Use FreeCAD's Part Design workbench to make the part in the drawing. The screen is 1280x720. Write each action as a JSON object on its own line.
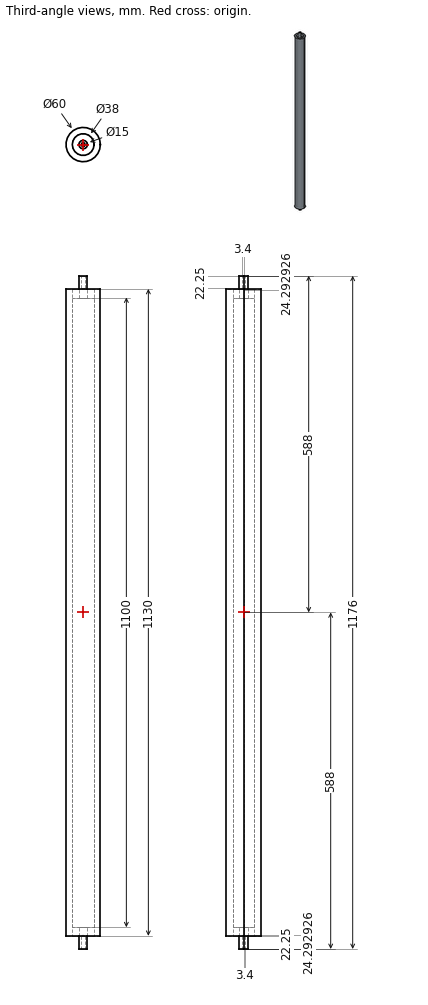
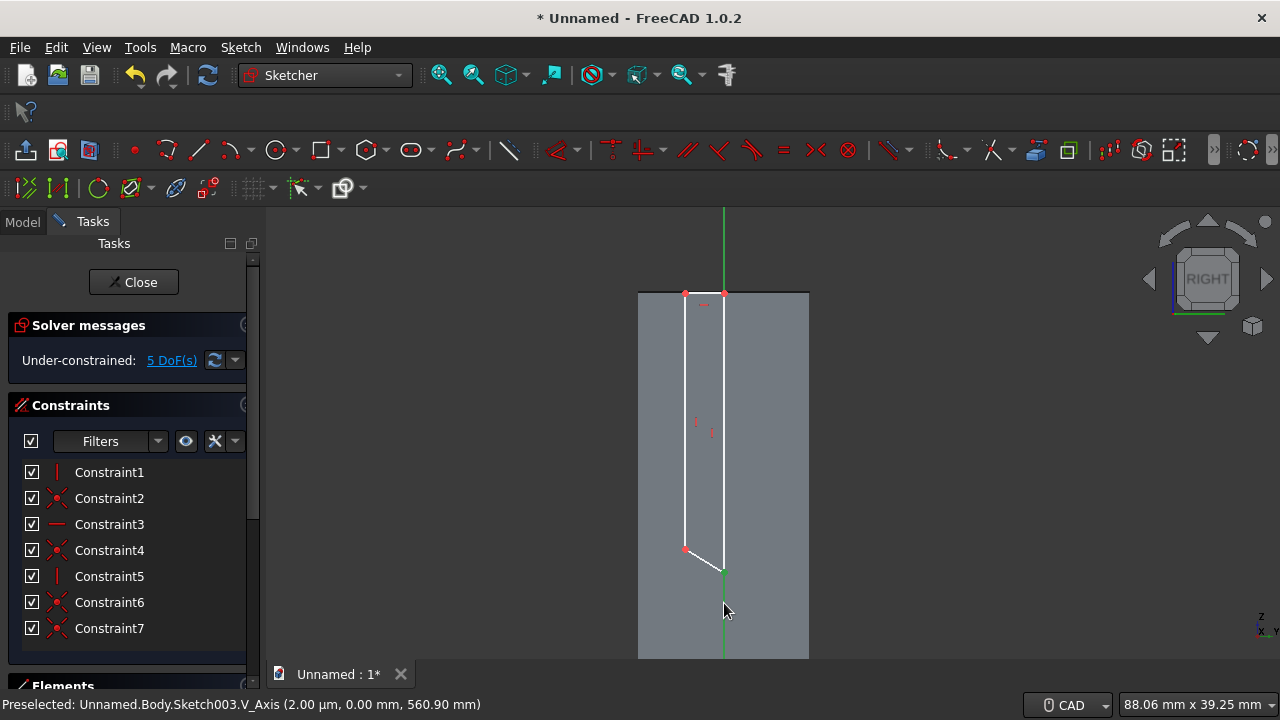
{"action": "left_click", "coordinate": [612, 150]}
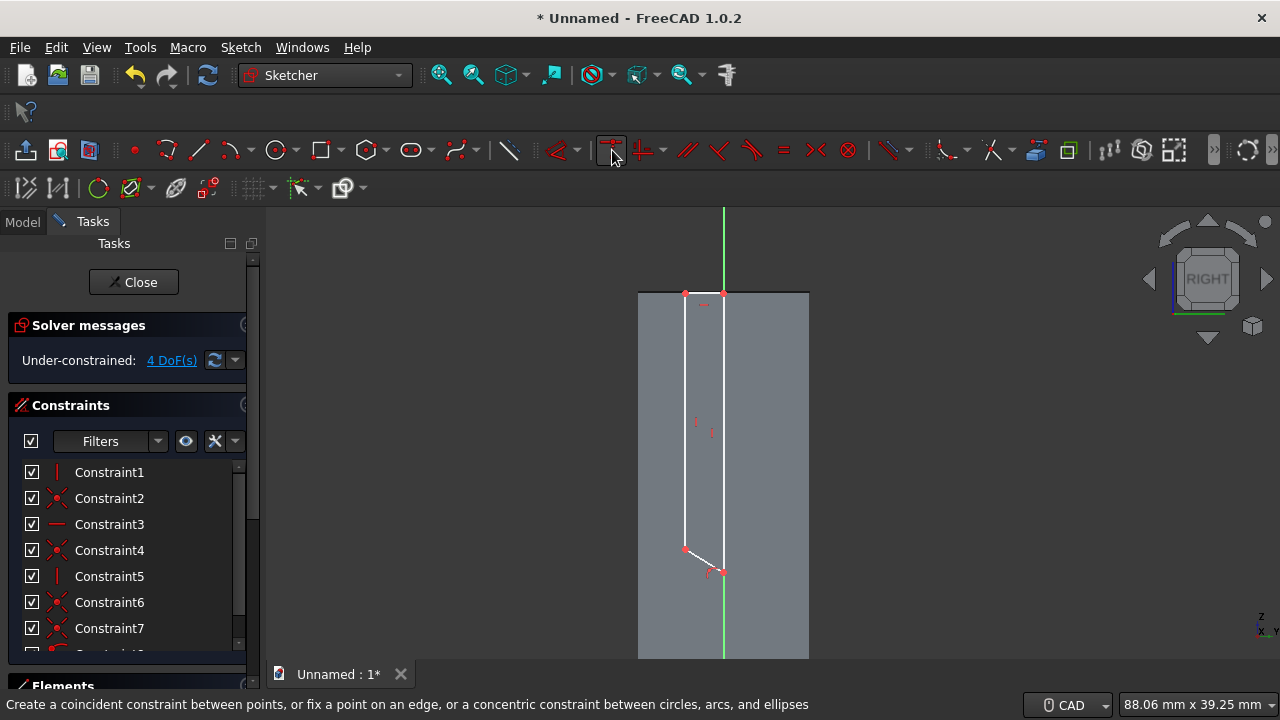
{"action": "key", "text": "d"}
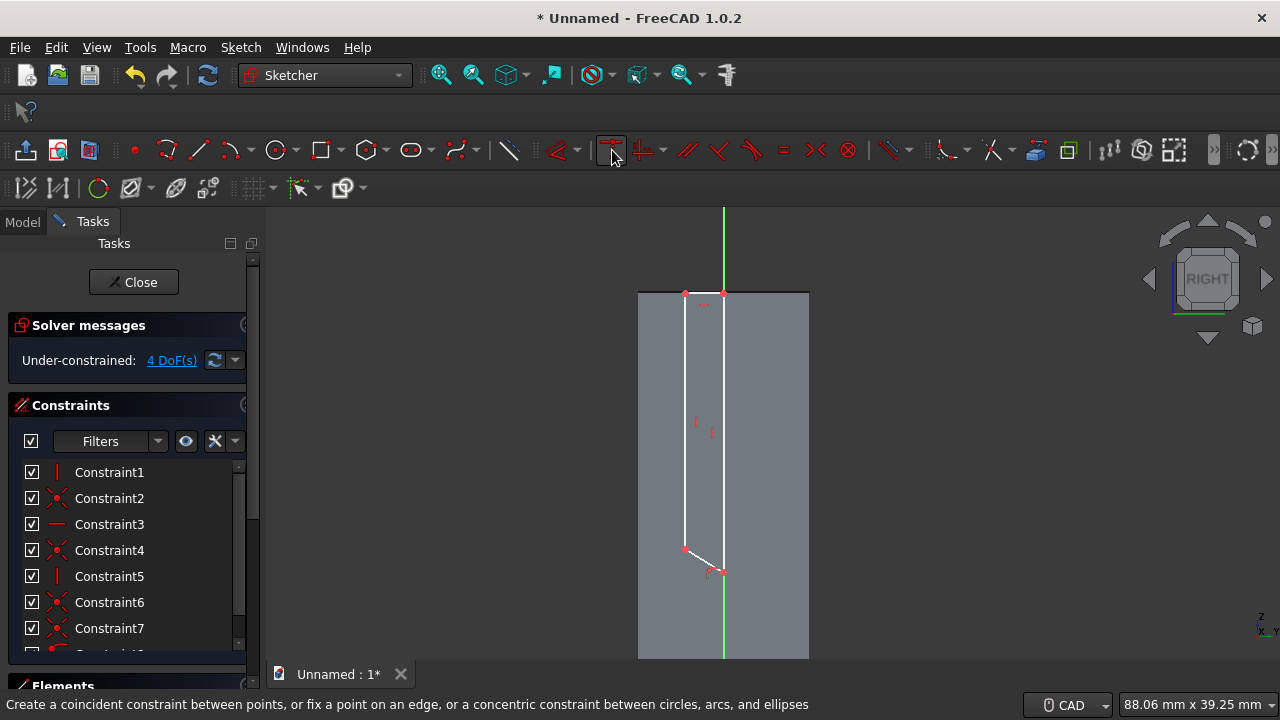
{"action": "left_click", "coordinate": [712, 293]}
{"action": "left_click", "coordinate": [704, 259]}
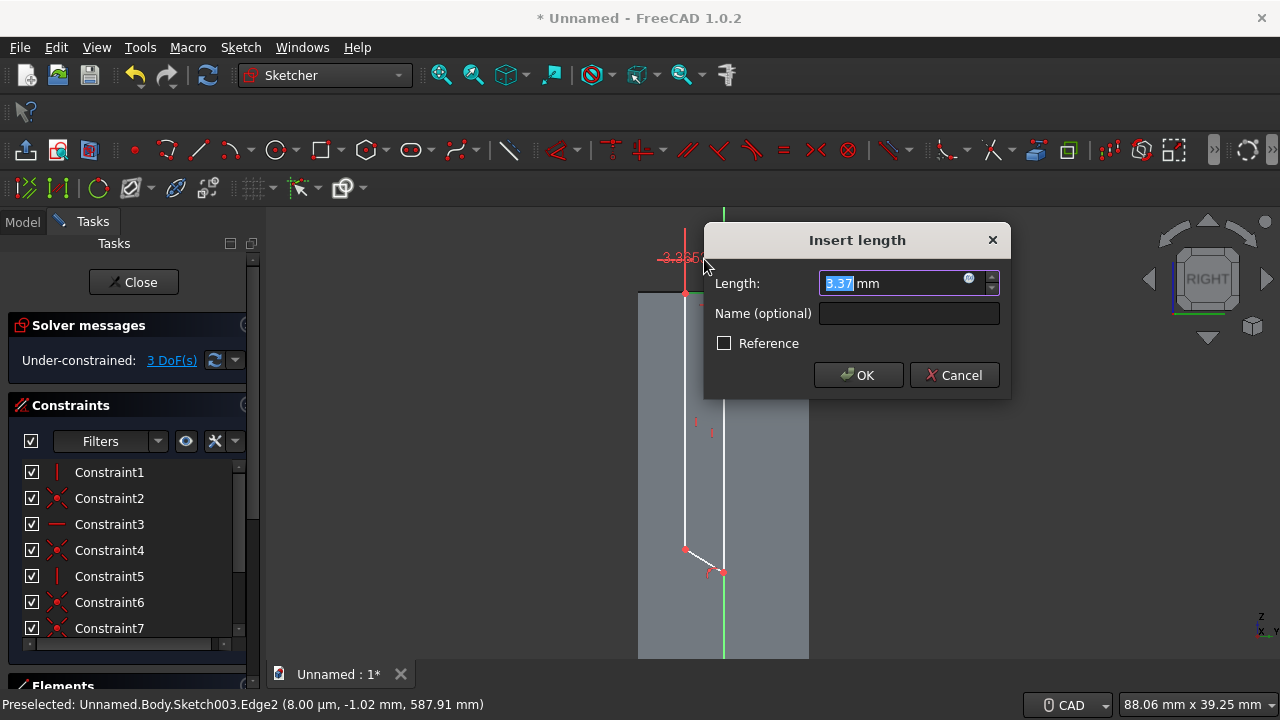
{"action": "type", "text": "3.4"}
{"action": "key", "text": "Return"}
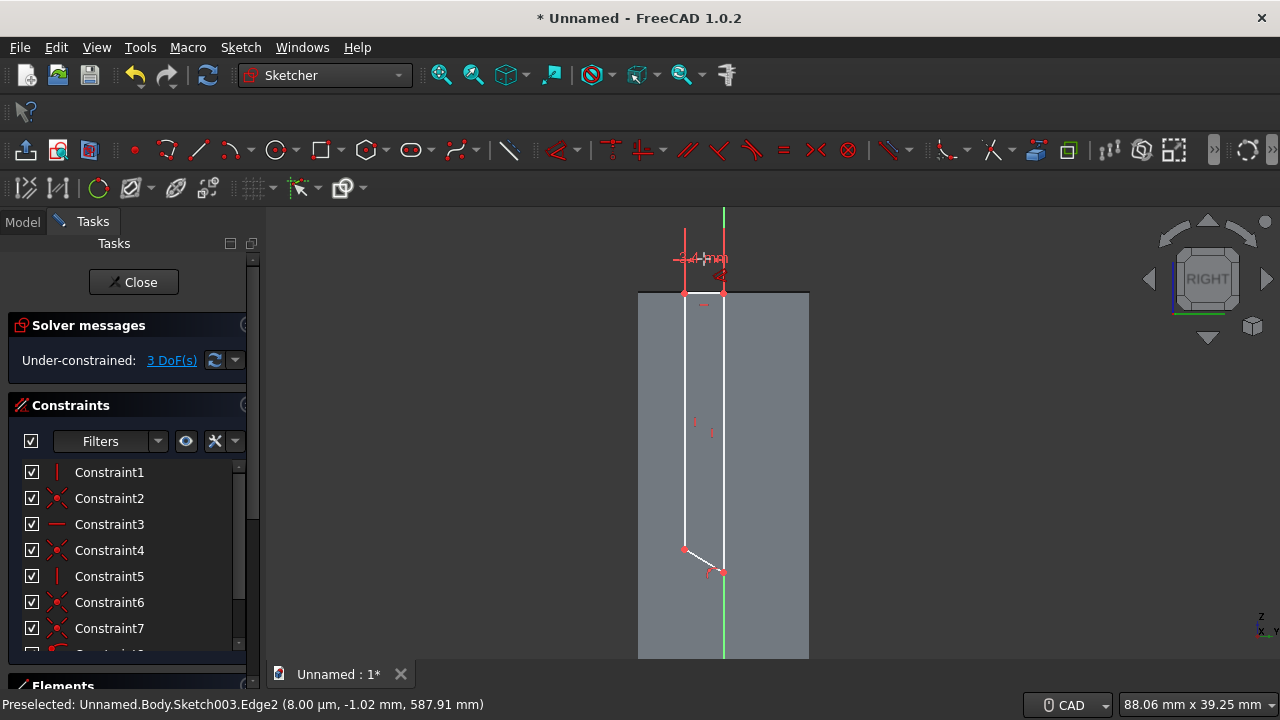
{"action": "left_click", "coordinate": [724, 293]}
{"action": "left_click", "coordinate": [758, 462]}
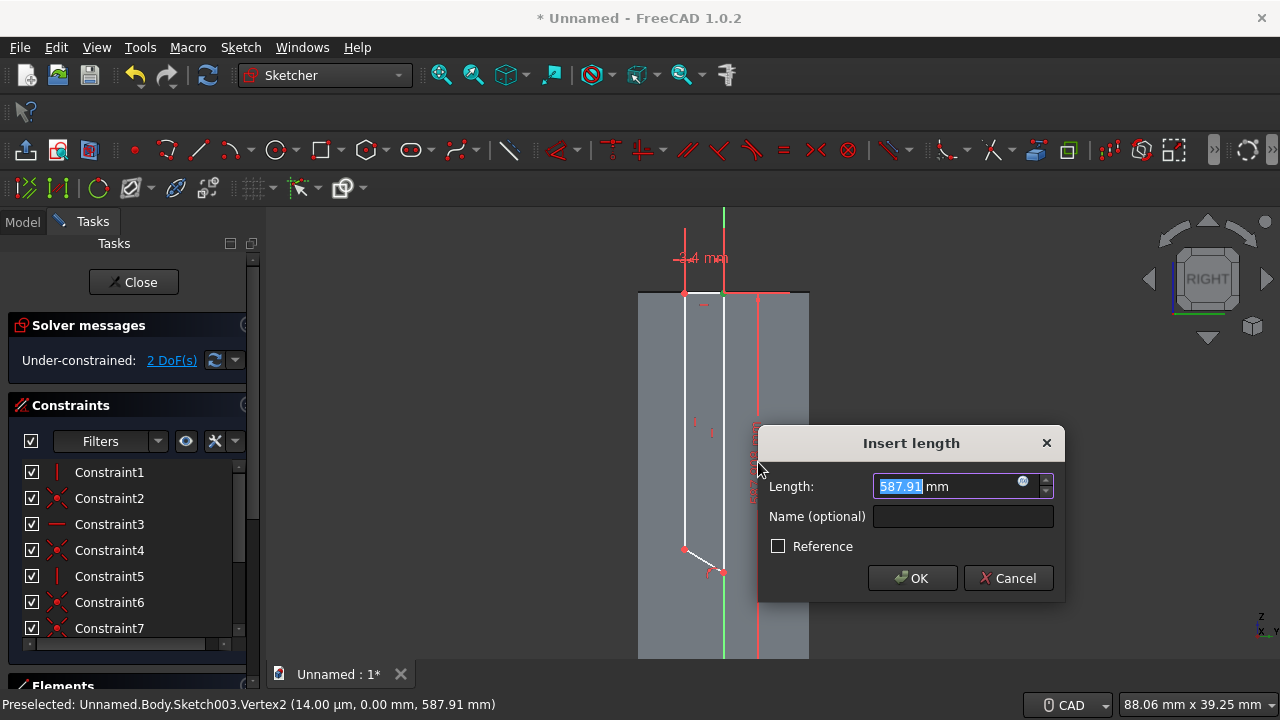
{"action": "type", "text": "588"}
{"action": "key", "text": "Return"}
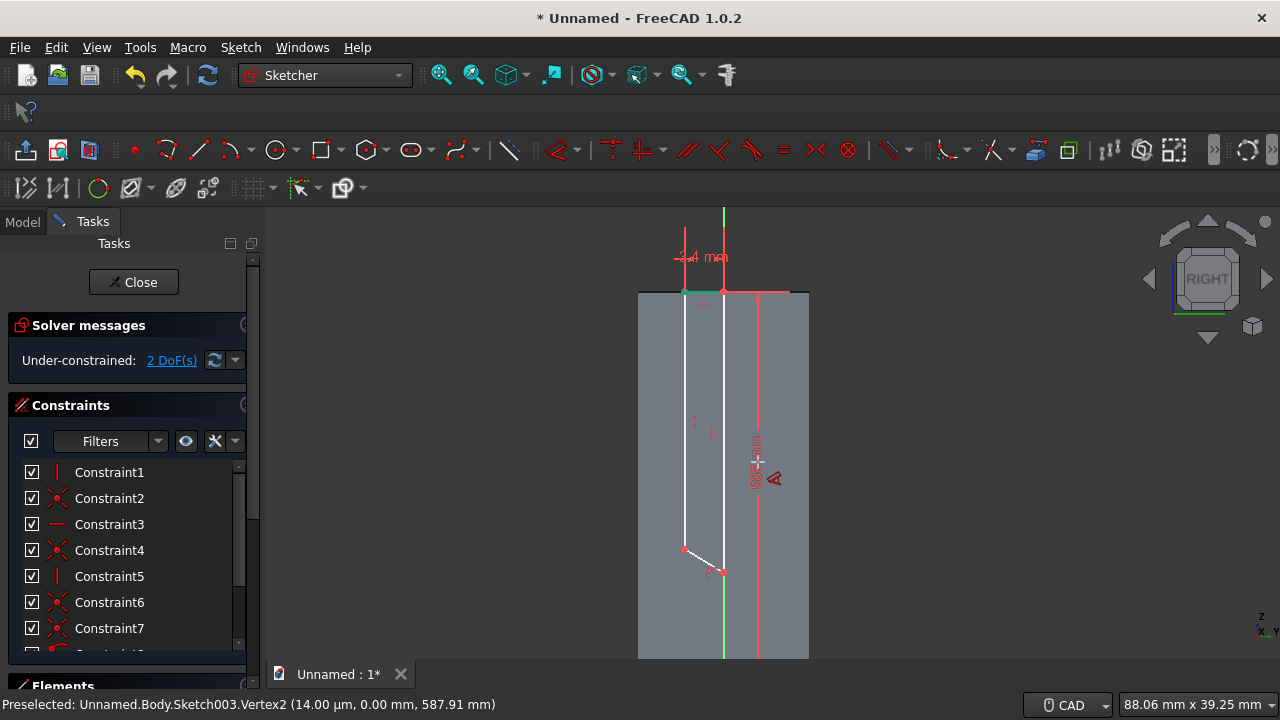
{"action": "left_click", "coordinate": [685, 369]}
{"action": "left_click", "coordinate": [651, 420]}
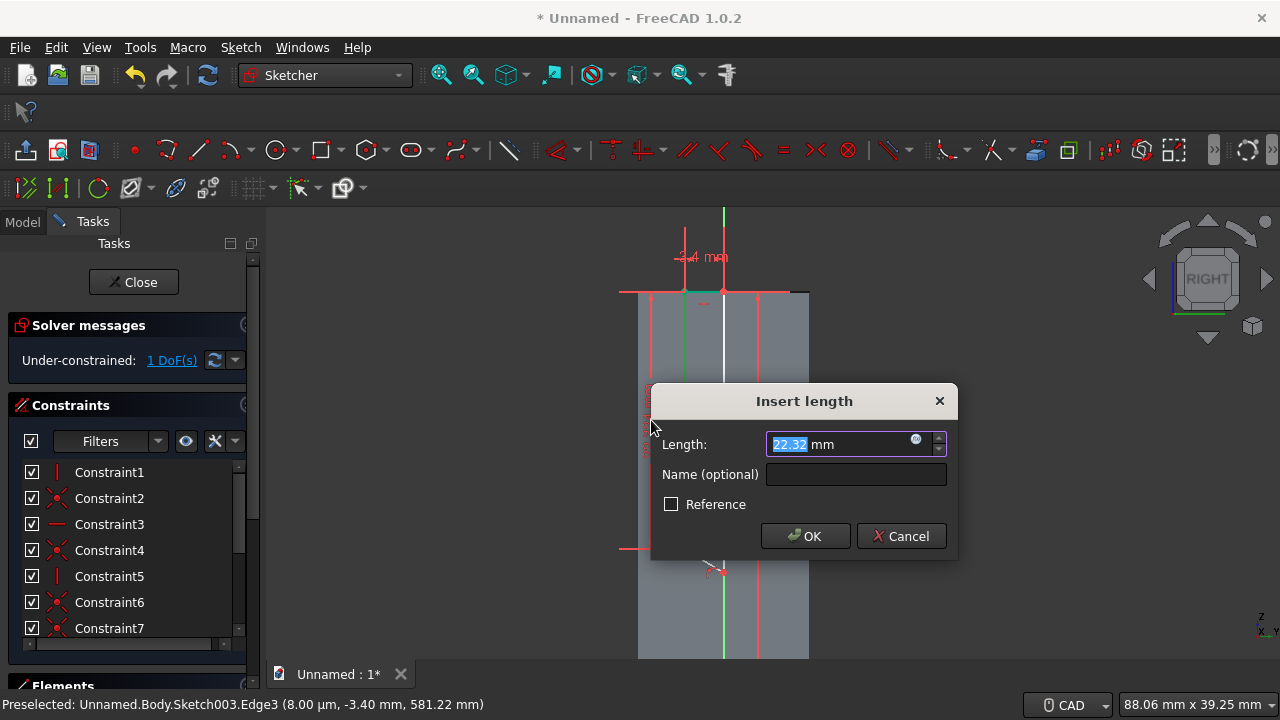
{"action": "type", "text": "22.25"}
{"action": "key", "text": "Return"}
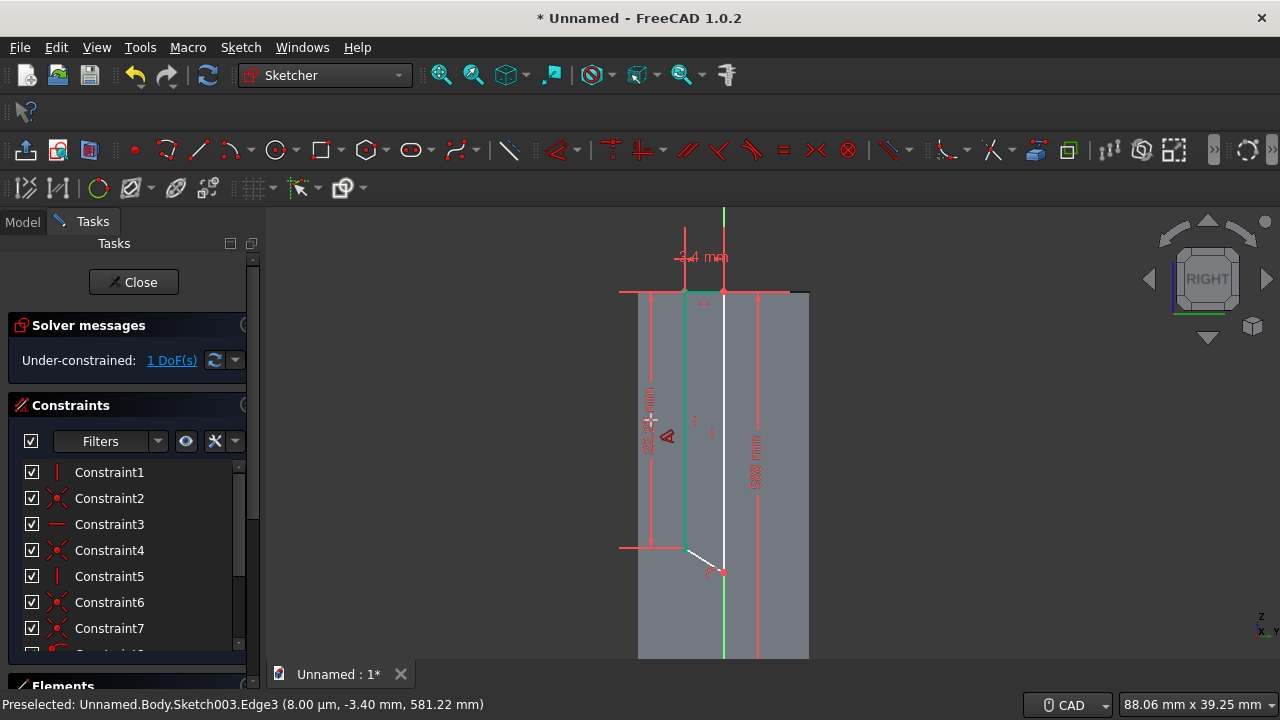
{"action": "left_click", "coordinate": [724, 489]}
{"action": "left_click", "coordinate": [758, 432]}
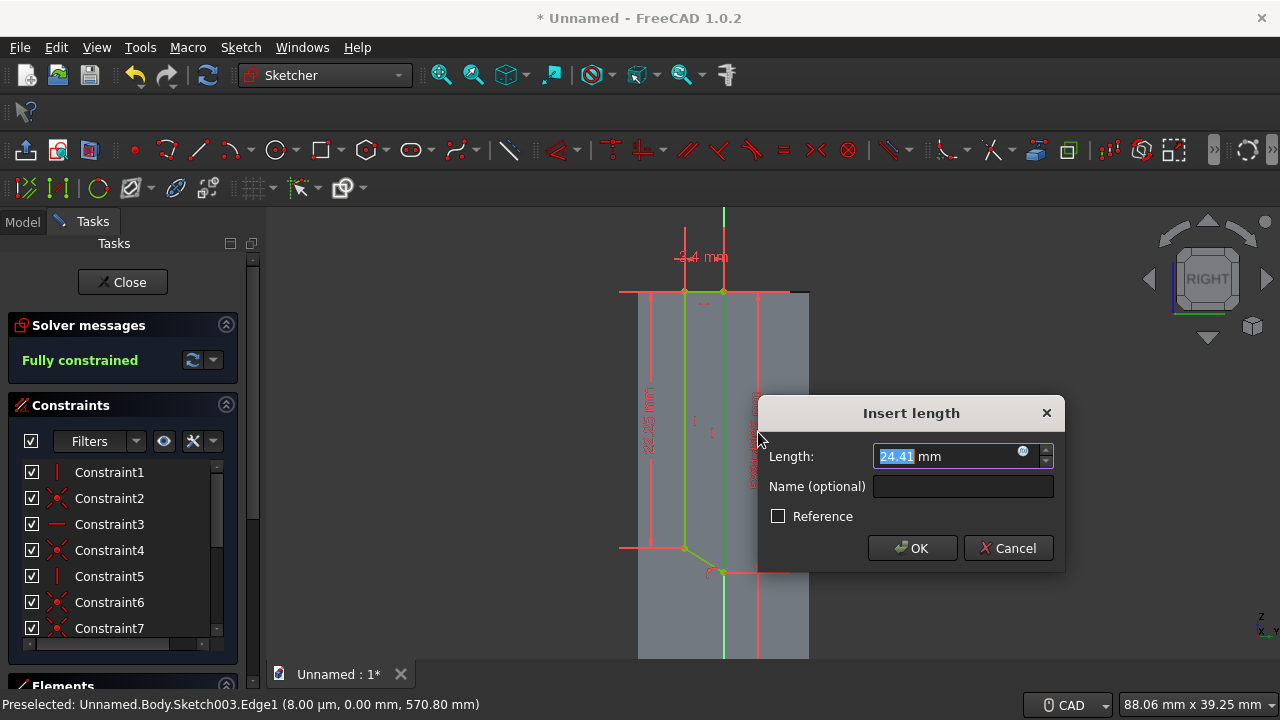
{"action": "type", "text": "24.292926"}
{"action": "key", "text": "Return"}
{"action": "key", "text": "Escape"}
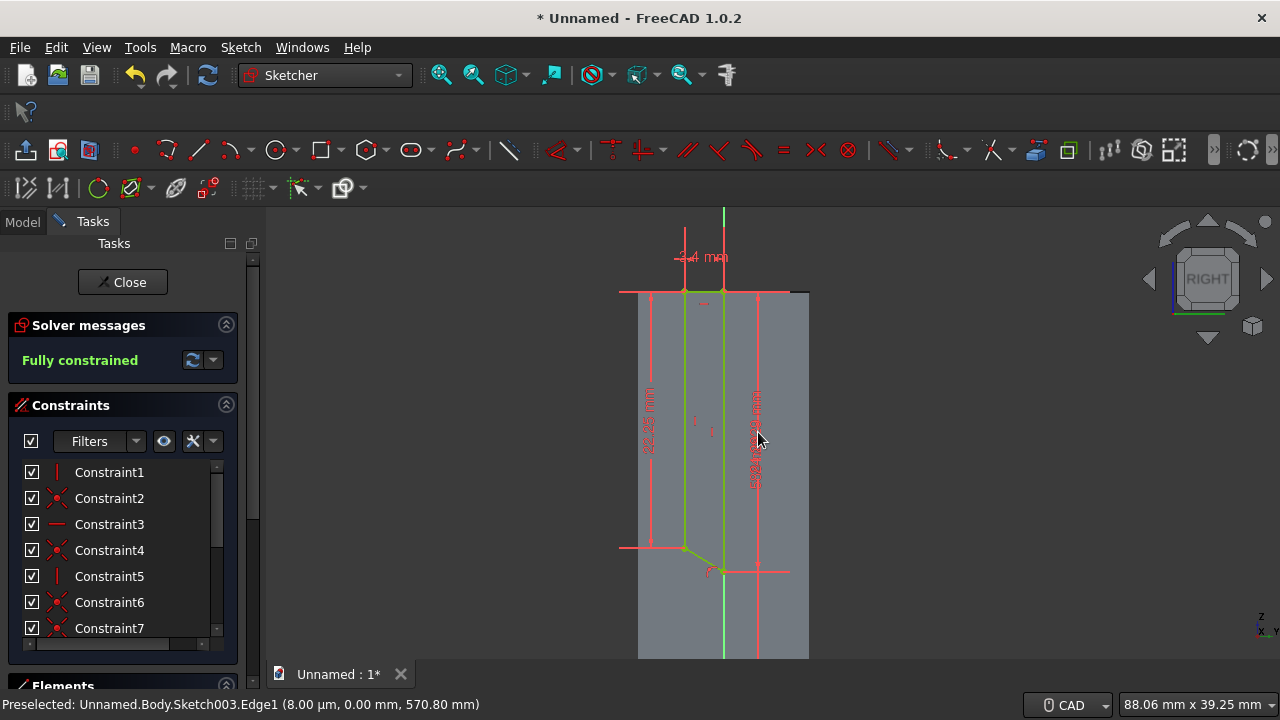
{"action": "left_click", "coordinate": [123, 282]}